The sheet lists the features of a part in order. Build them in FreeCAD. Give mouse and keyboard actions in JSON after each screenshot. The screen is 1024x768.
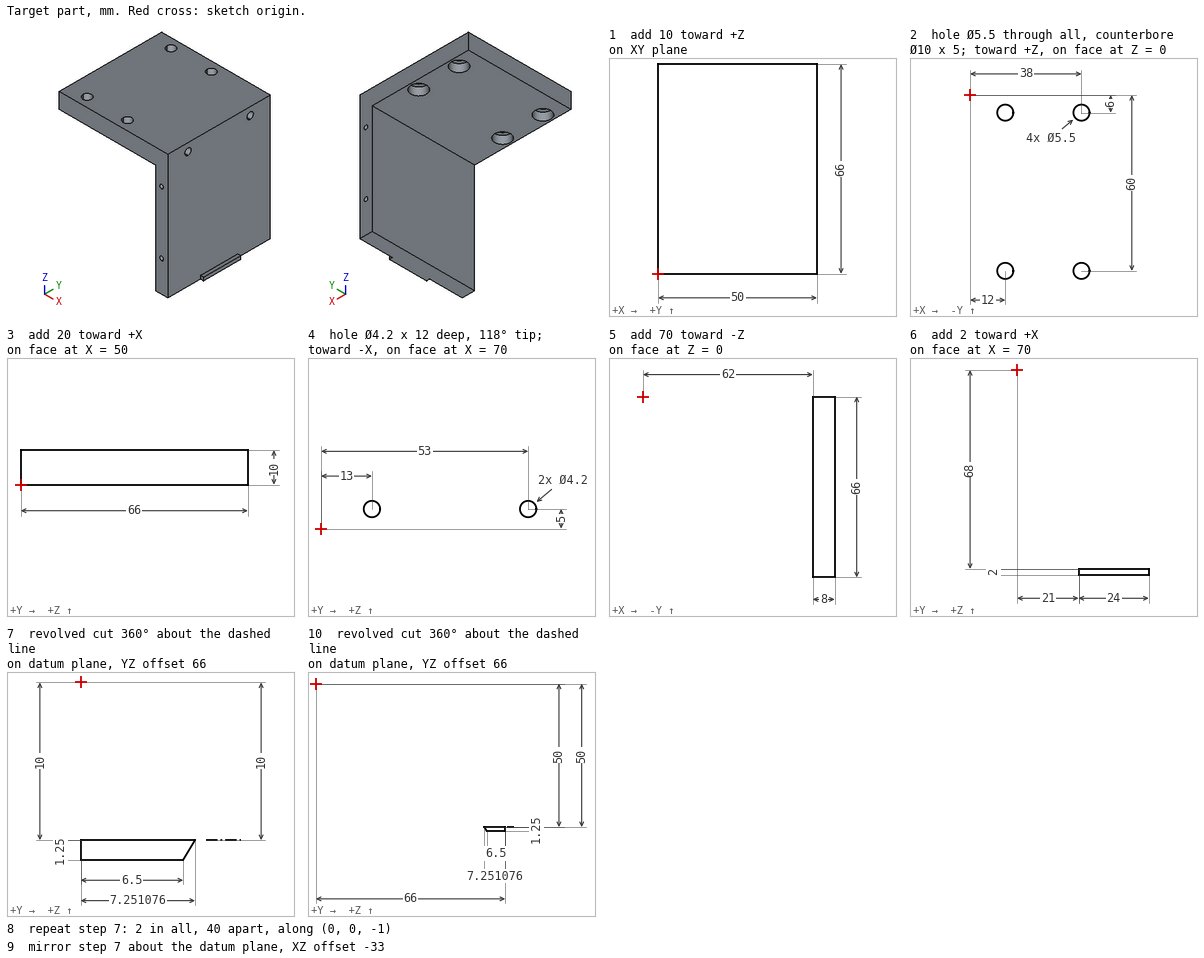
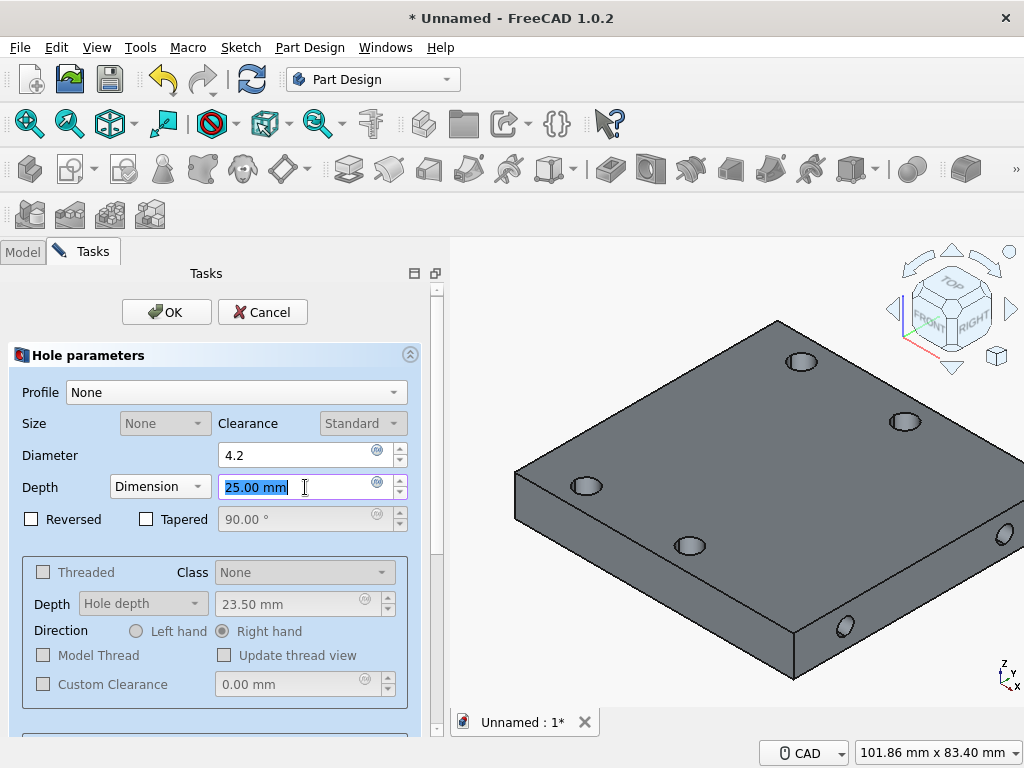
{"action": "type", "text": "12"}
{"action": "key", "text": "Tab"}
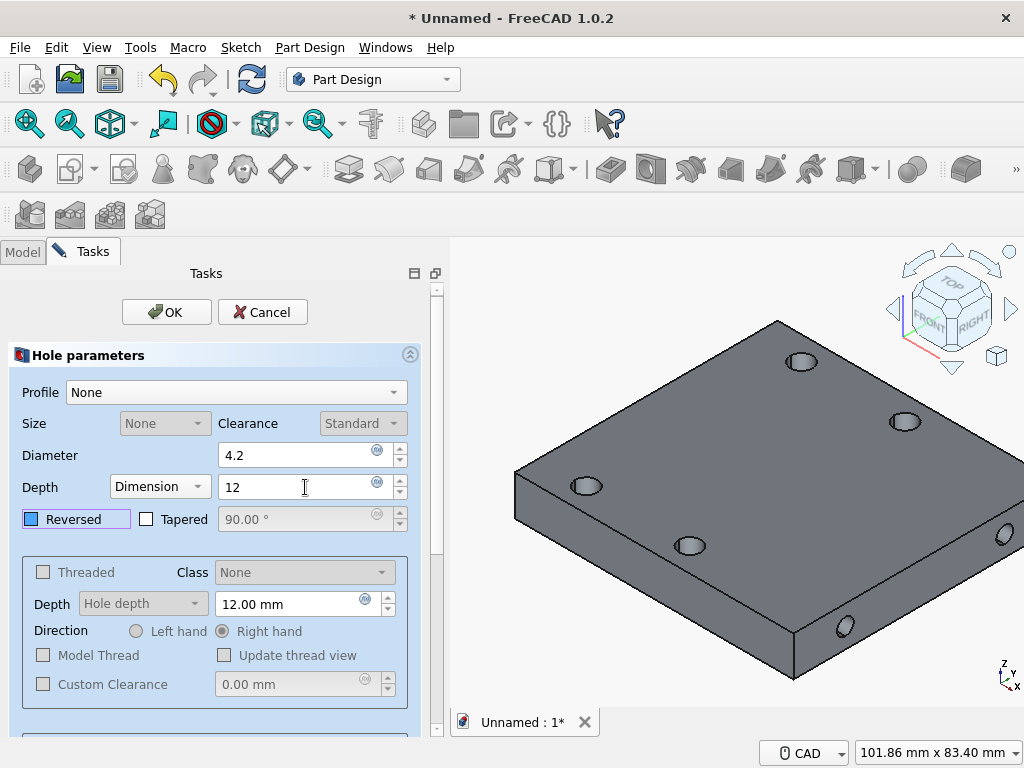
{"action": "left_click", "coordinate": [167, 312]}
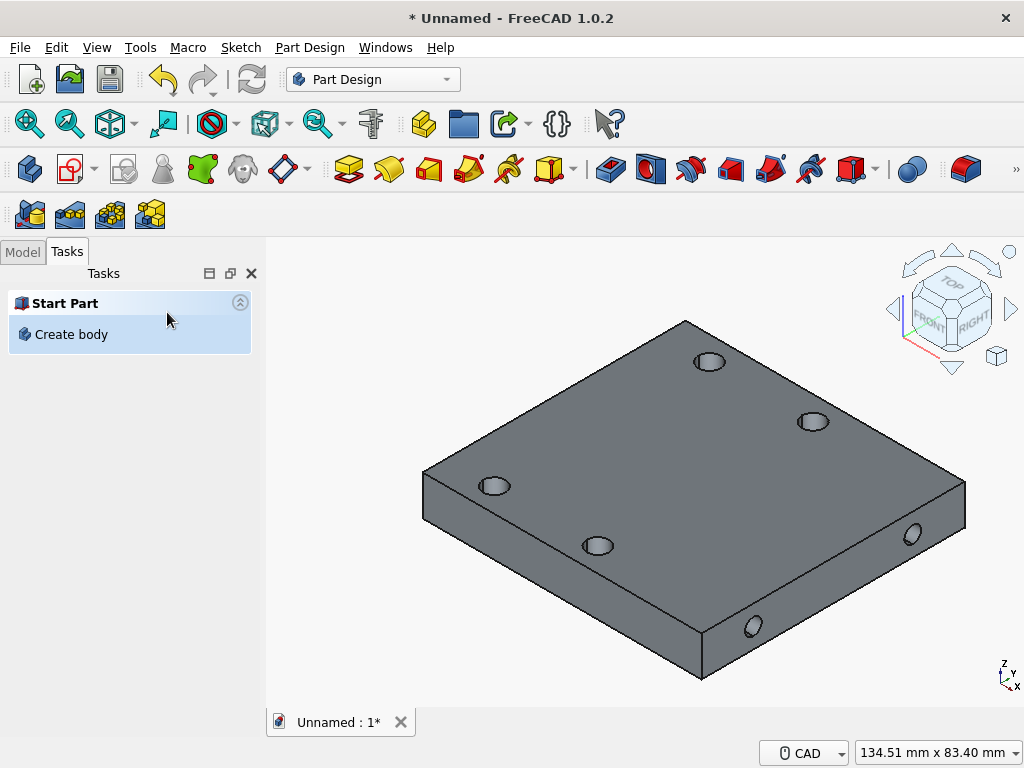
{"action": "key", "text": "5"}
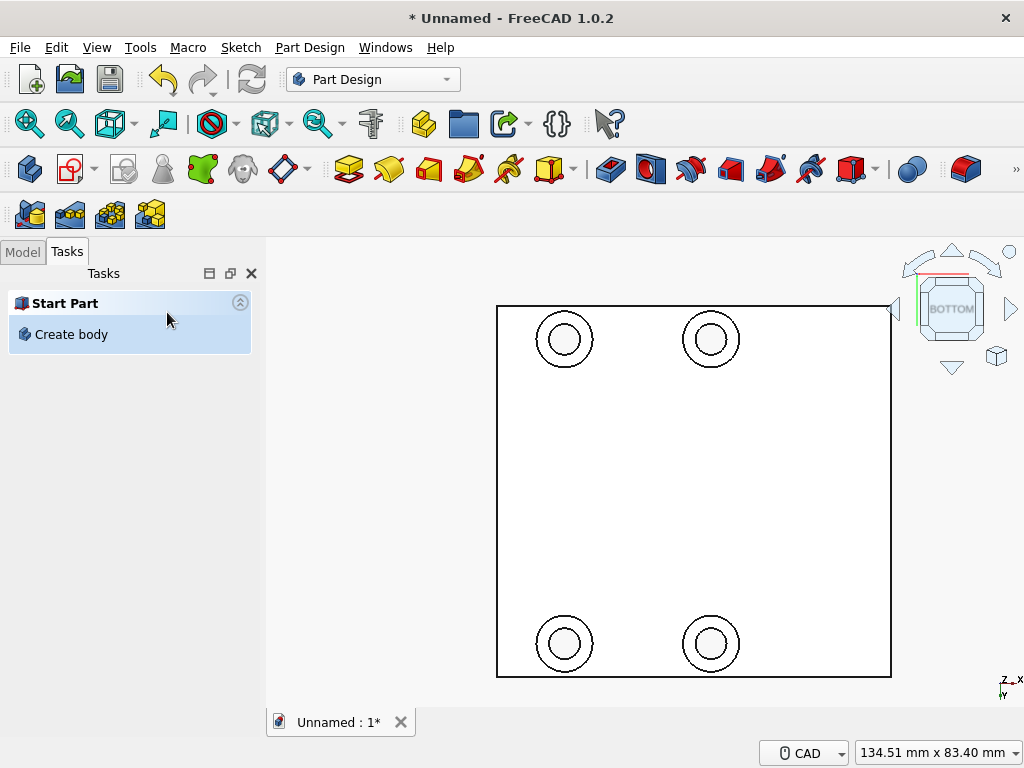
{"action": "left_click", "coordinate": [638, 491]}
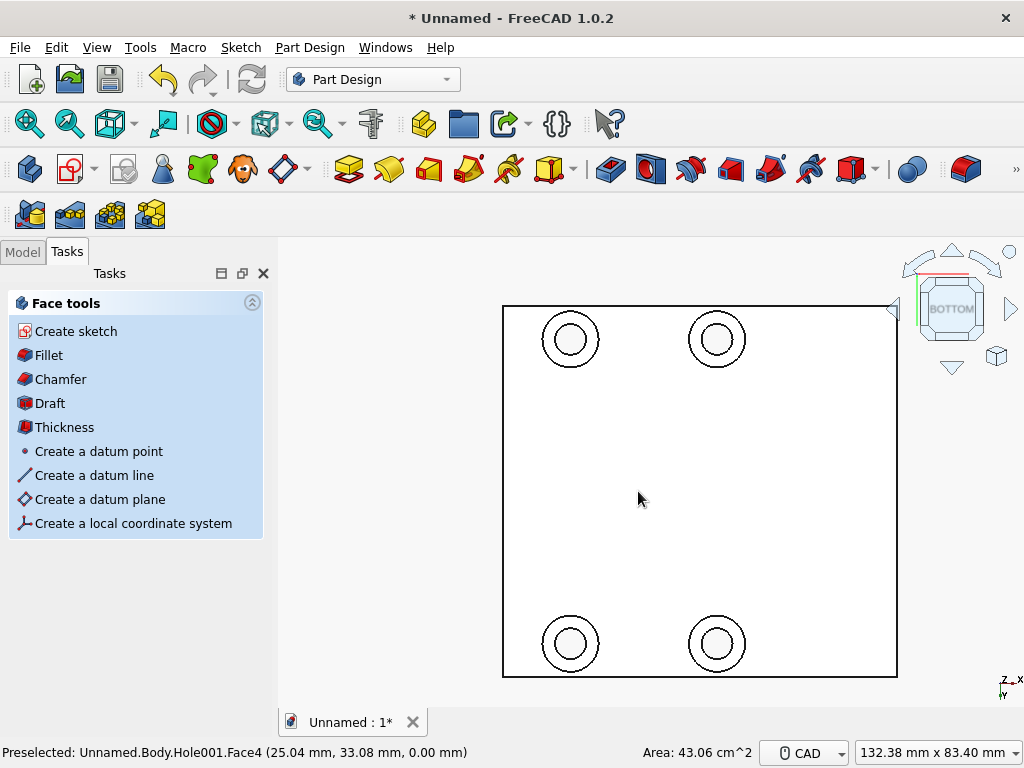
{"action": "left_click", "coordinate": [70, 170]}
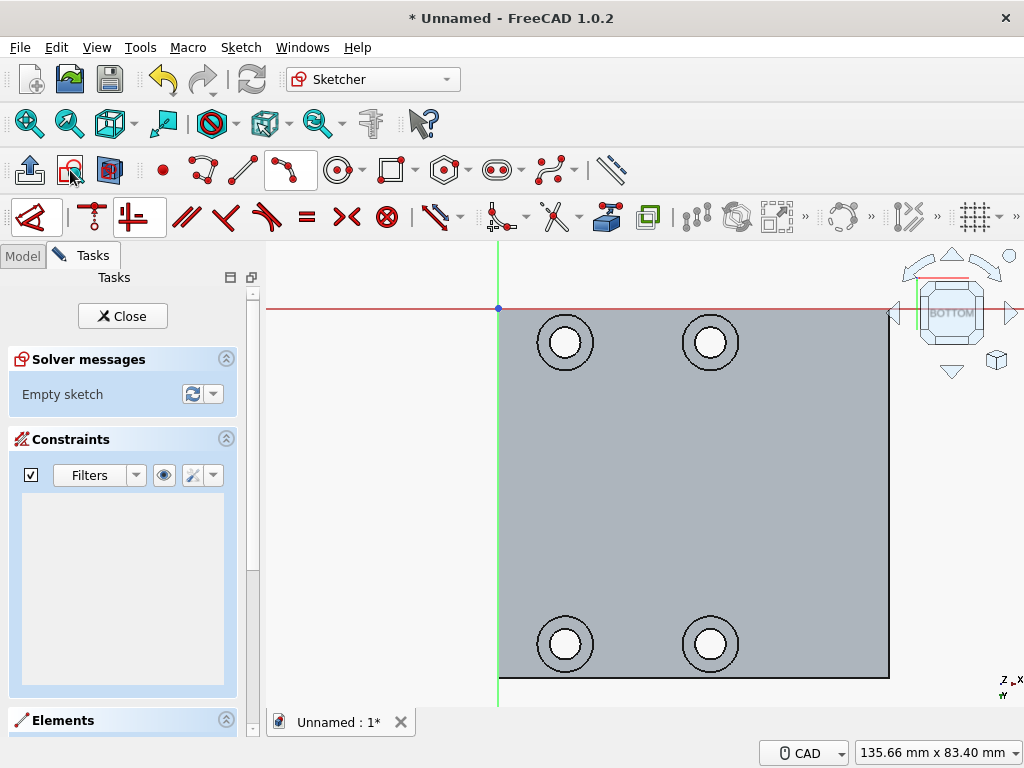
{"action": "scroll", "coordinate": [294, 387], "scroll_direction": "down", "scroll_amount": 1}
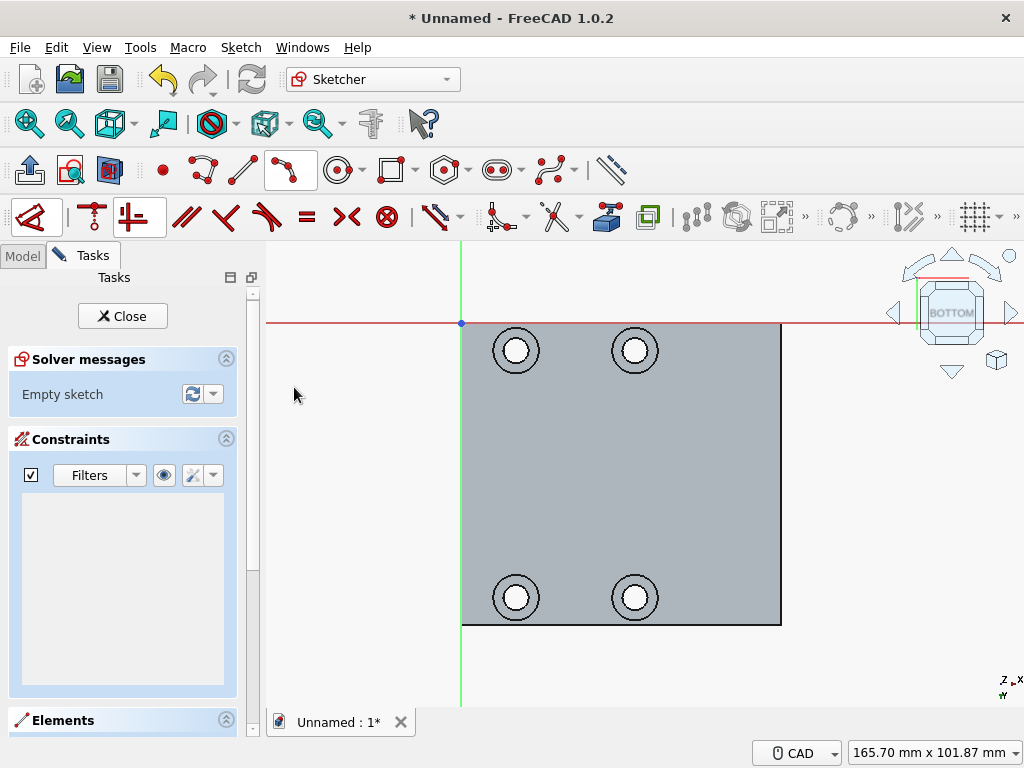
{"action": "left_click", "coordinate": [392, 170]}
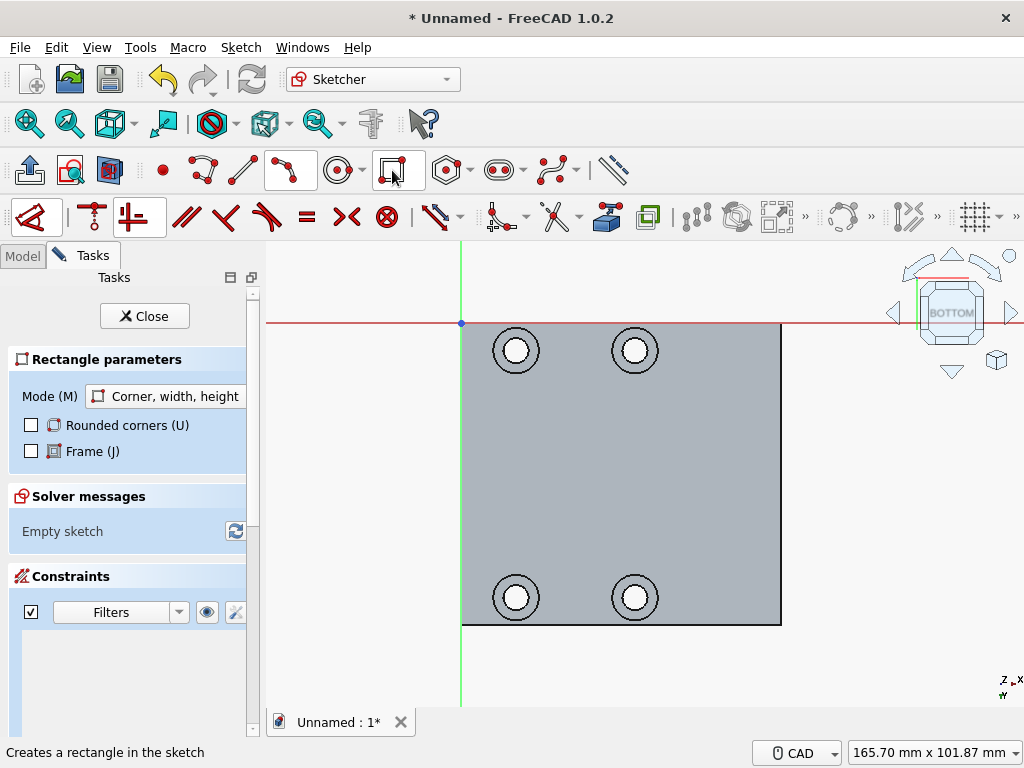
{"action": "left_click", "coordinate": [745, 323]}
{"action": "left_click", "coordinate": [781, 625]}
{"action": "key", "text": "Escape"}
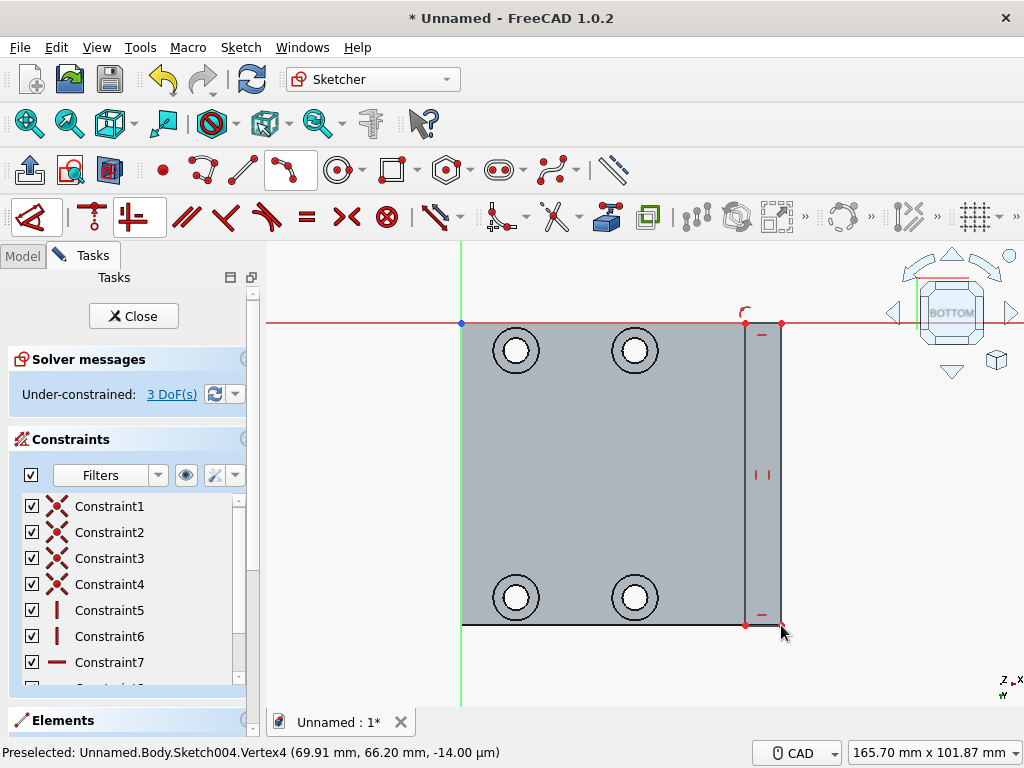
{"action": "scroll", "coordinate": [756, 626], "scroll_direction": "up", "scroll_amount": 2}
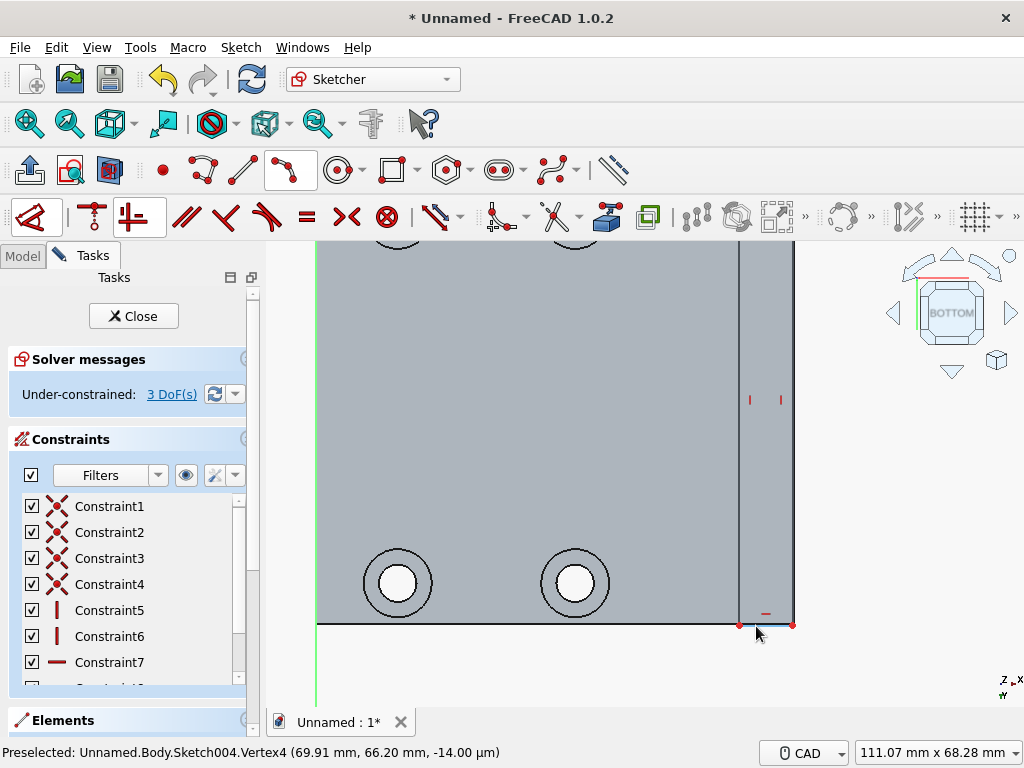
{"action": "left_click", "coordinate": [755, 626]}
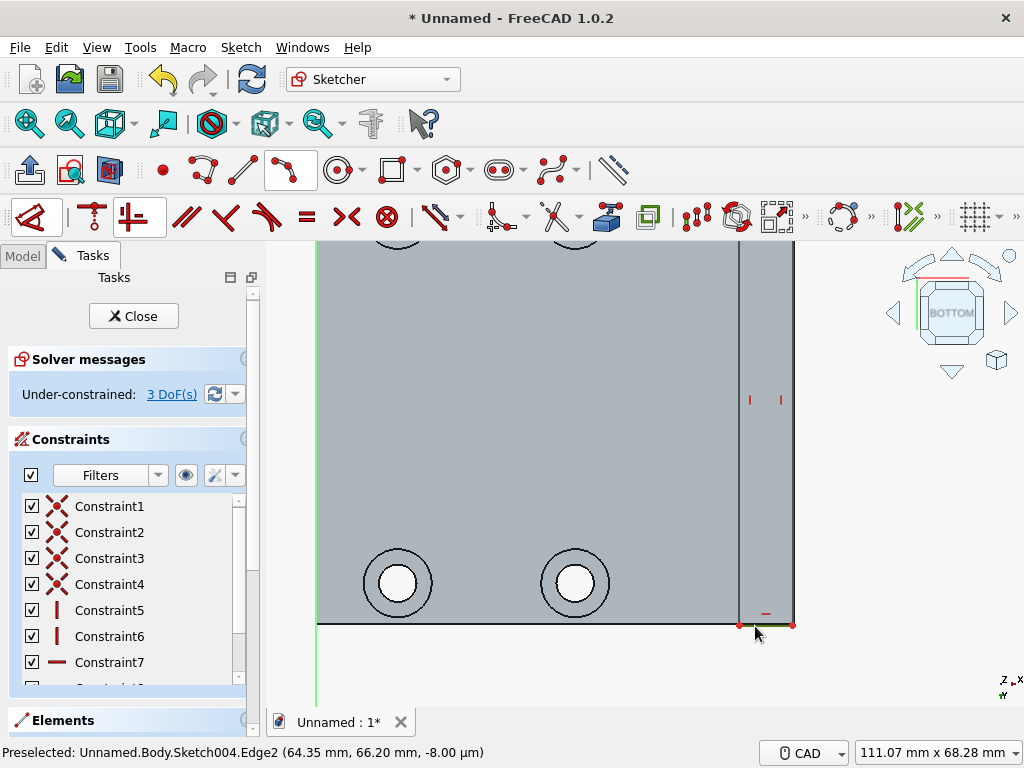
{"action": "key", "text": "l"}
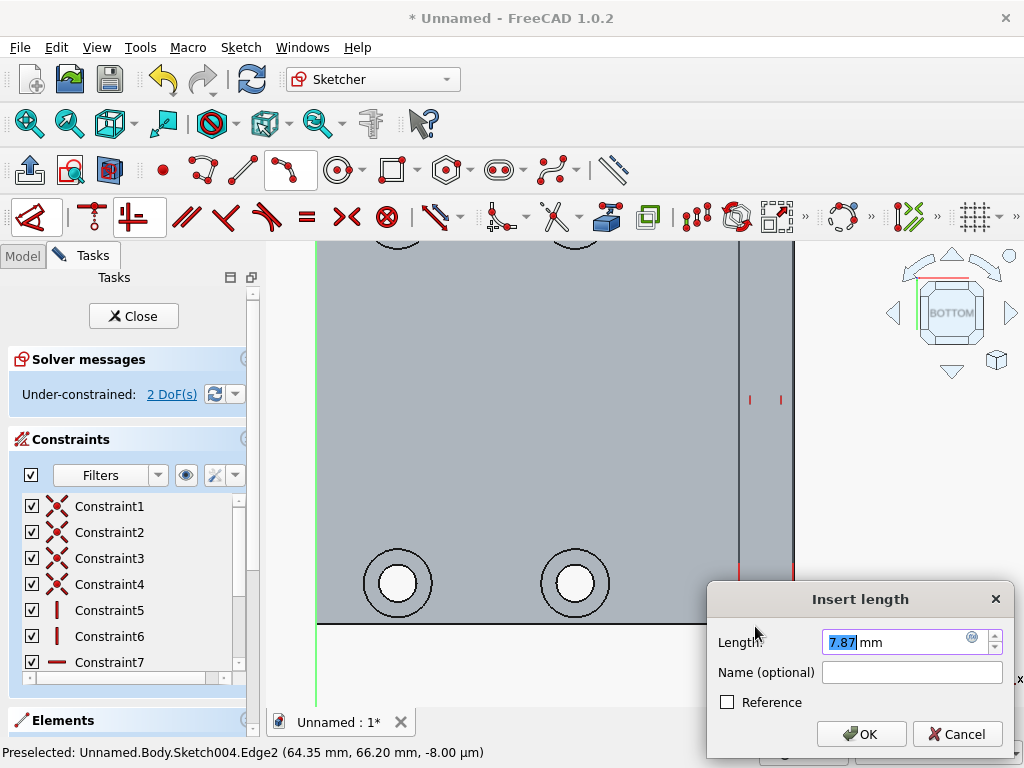
{"action": "type", "text": "8"}
{"action": "key", "text": "Return"}